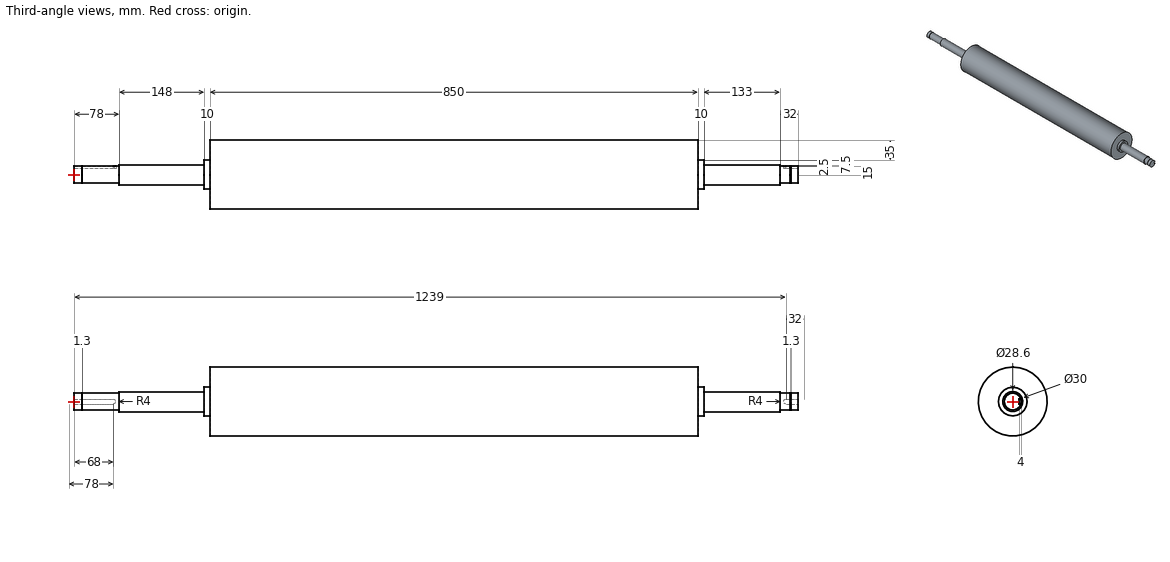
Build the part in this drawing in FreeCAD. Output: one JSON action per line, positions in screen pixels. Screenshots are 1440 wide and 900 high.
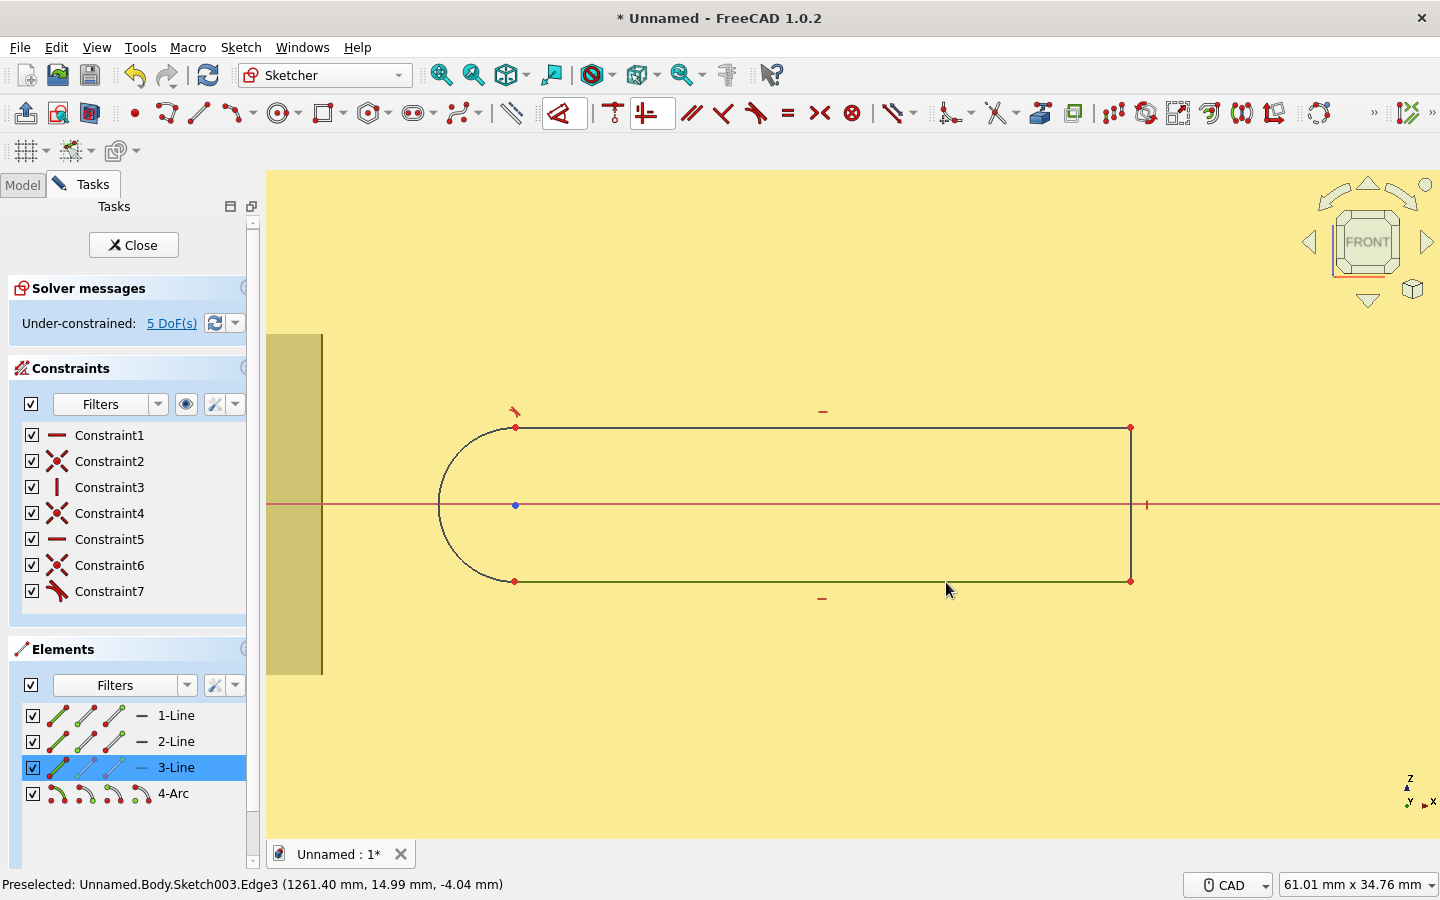
{"action": "left_click", "coordinate": [453, 460]}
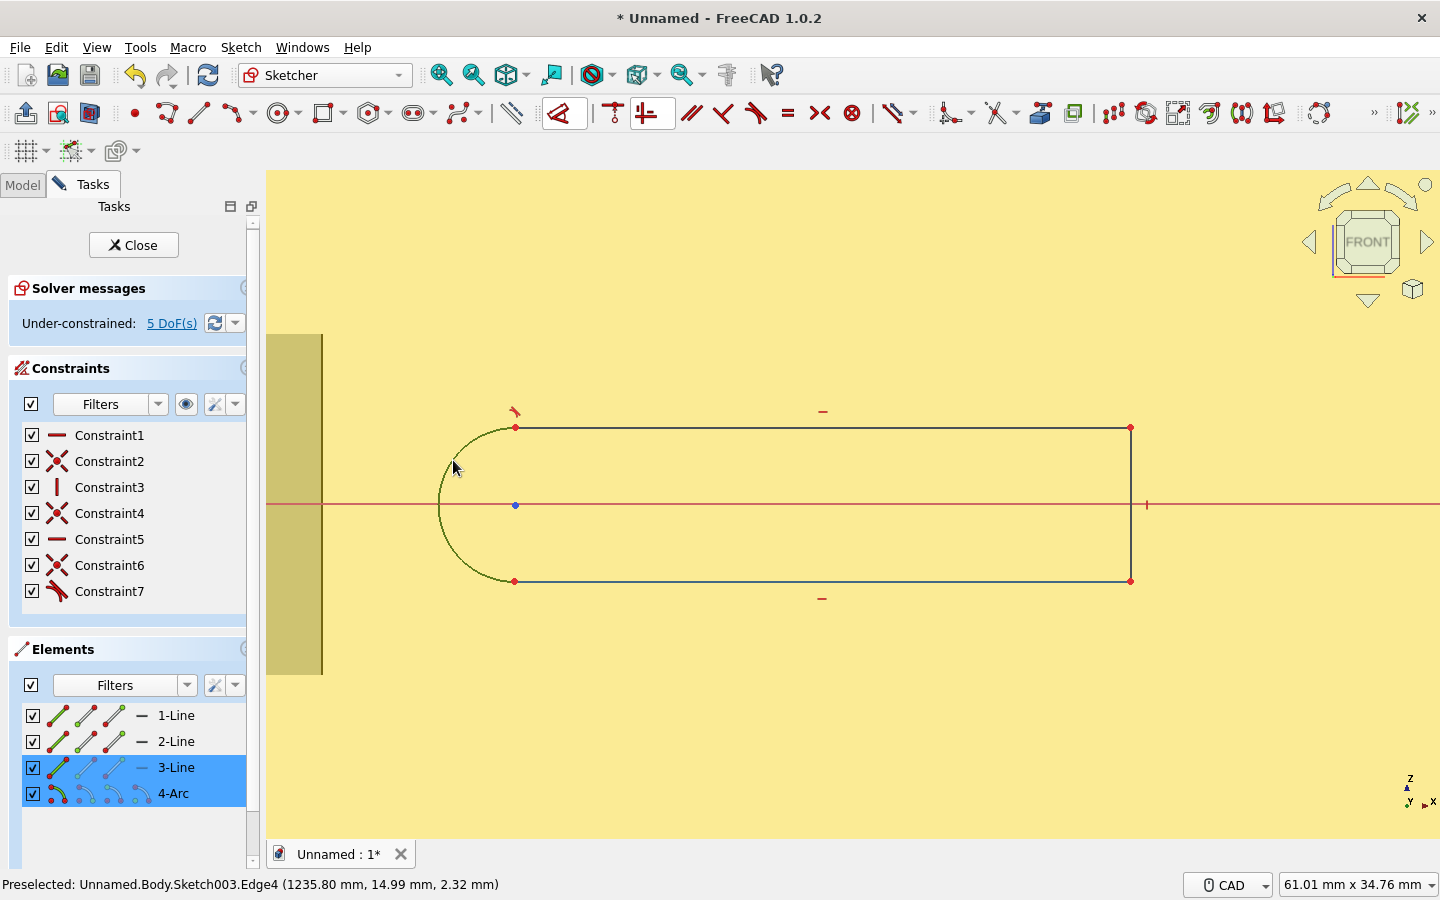
{"action": "left_click", "coordinate": [756, 114]}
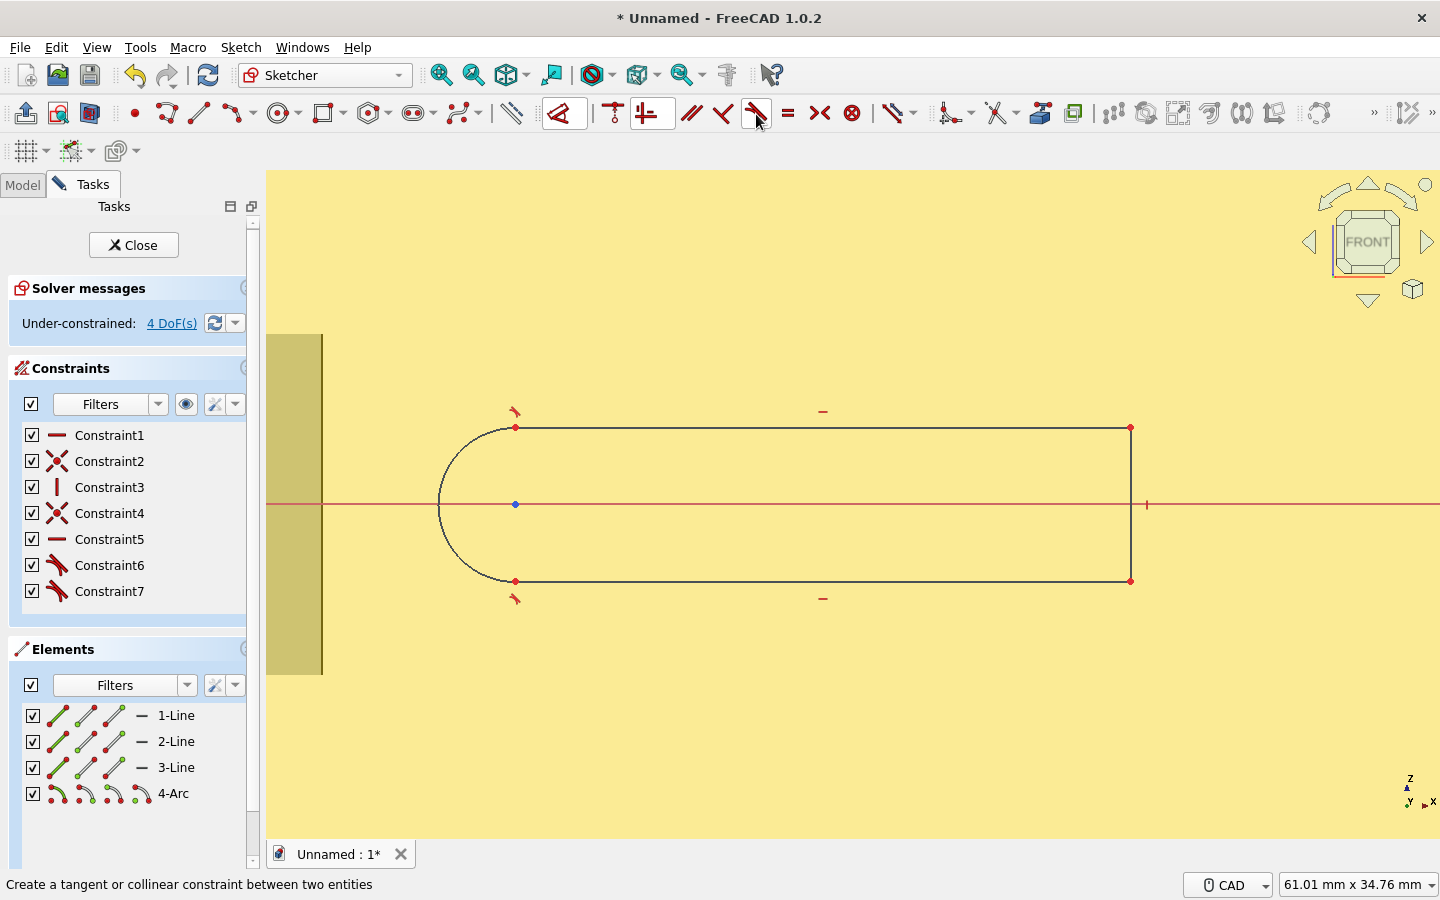
{"action": "left_click", "coordinate": [515, 505]}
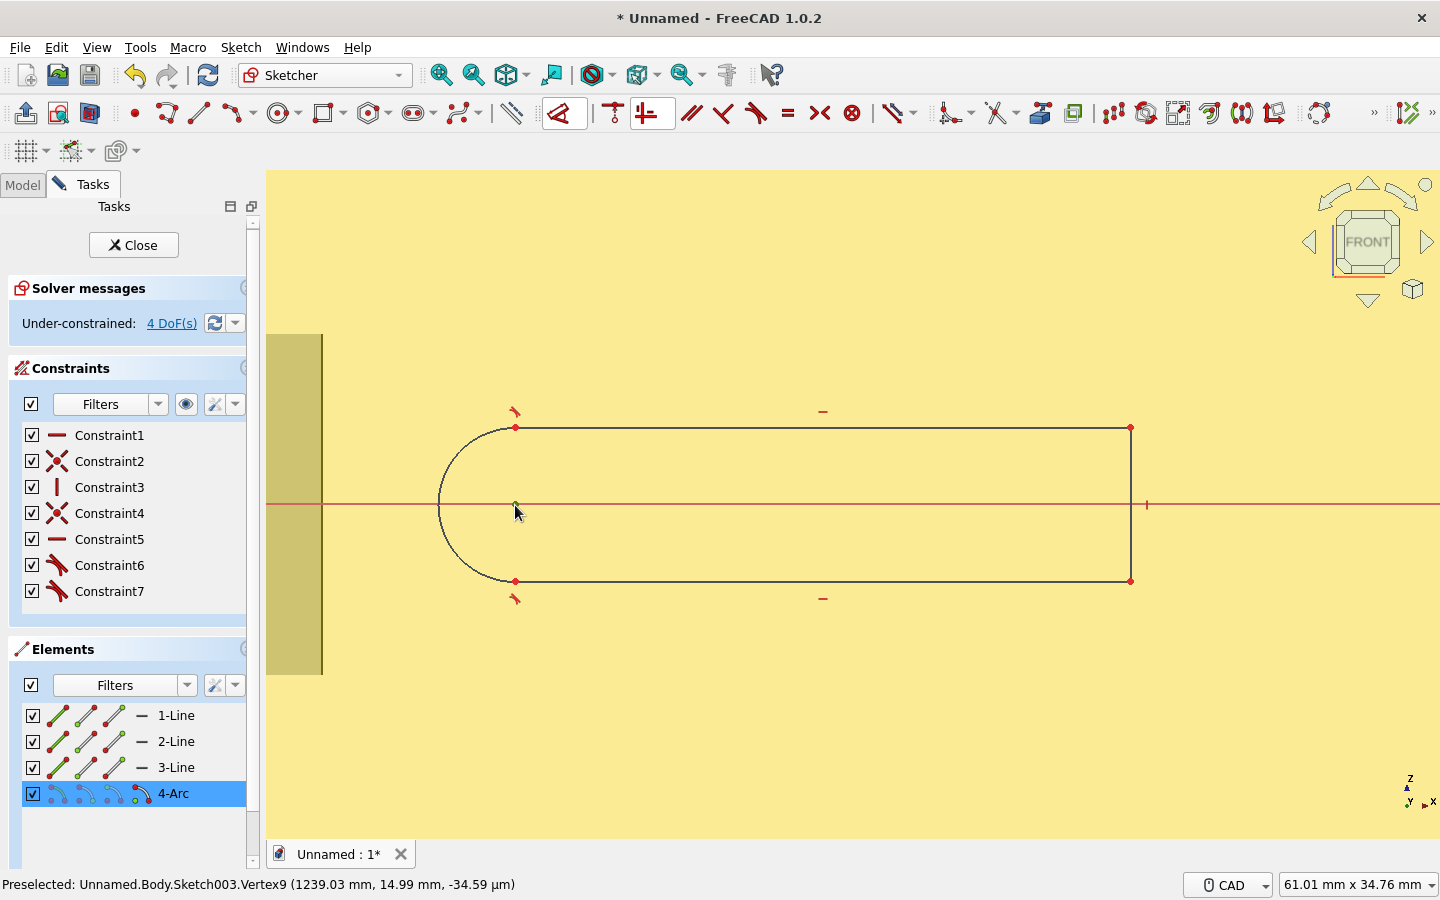
{"action": "left_click", "coordinate": [364, 504]}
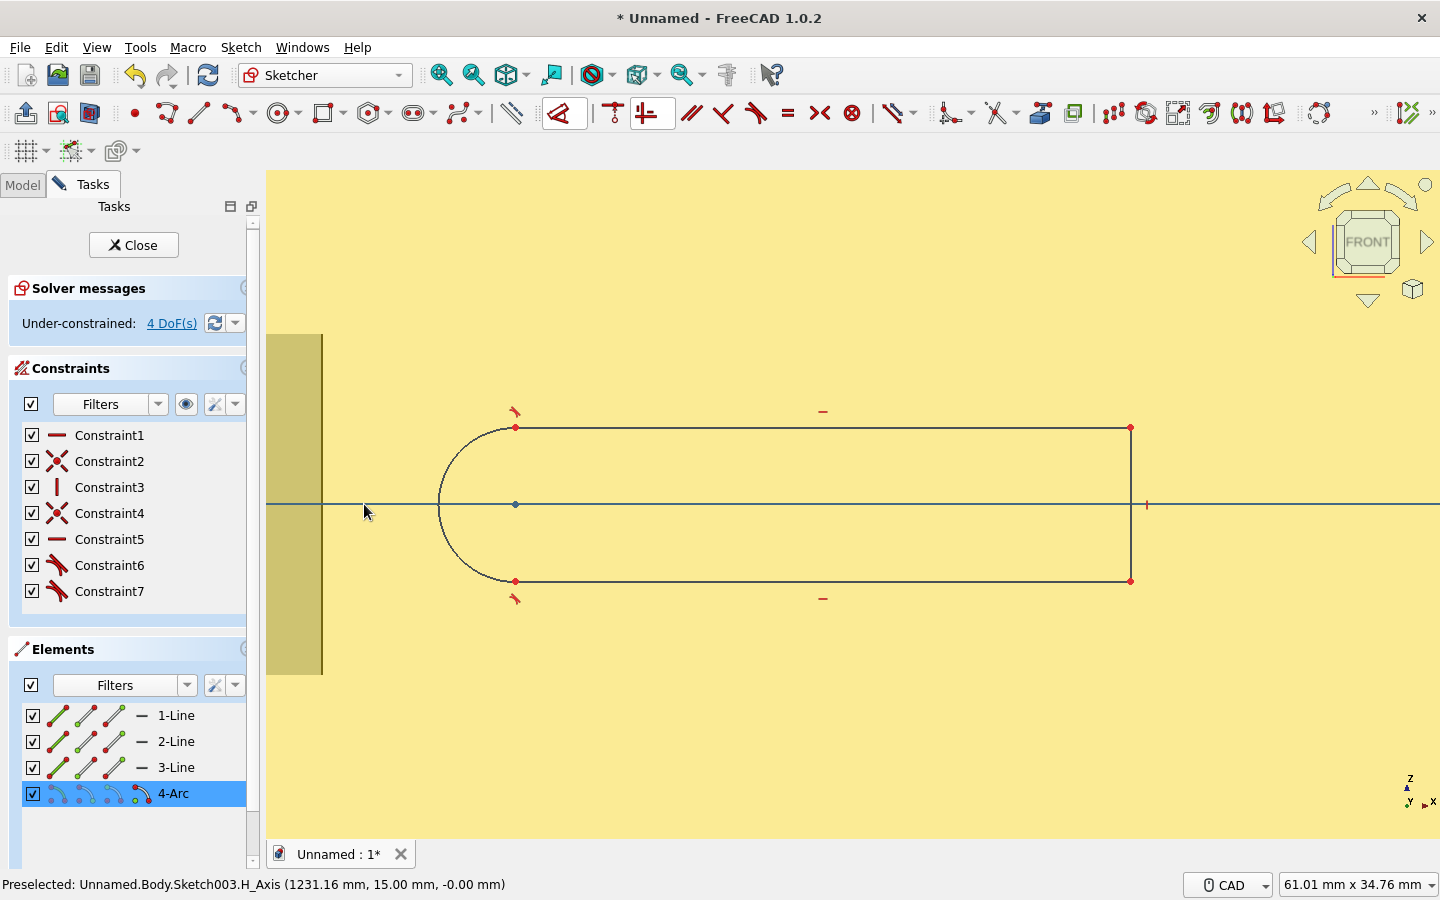
{"action": "left_click", "coordinate": [614, 114]}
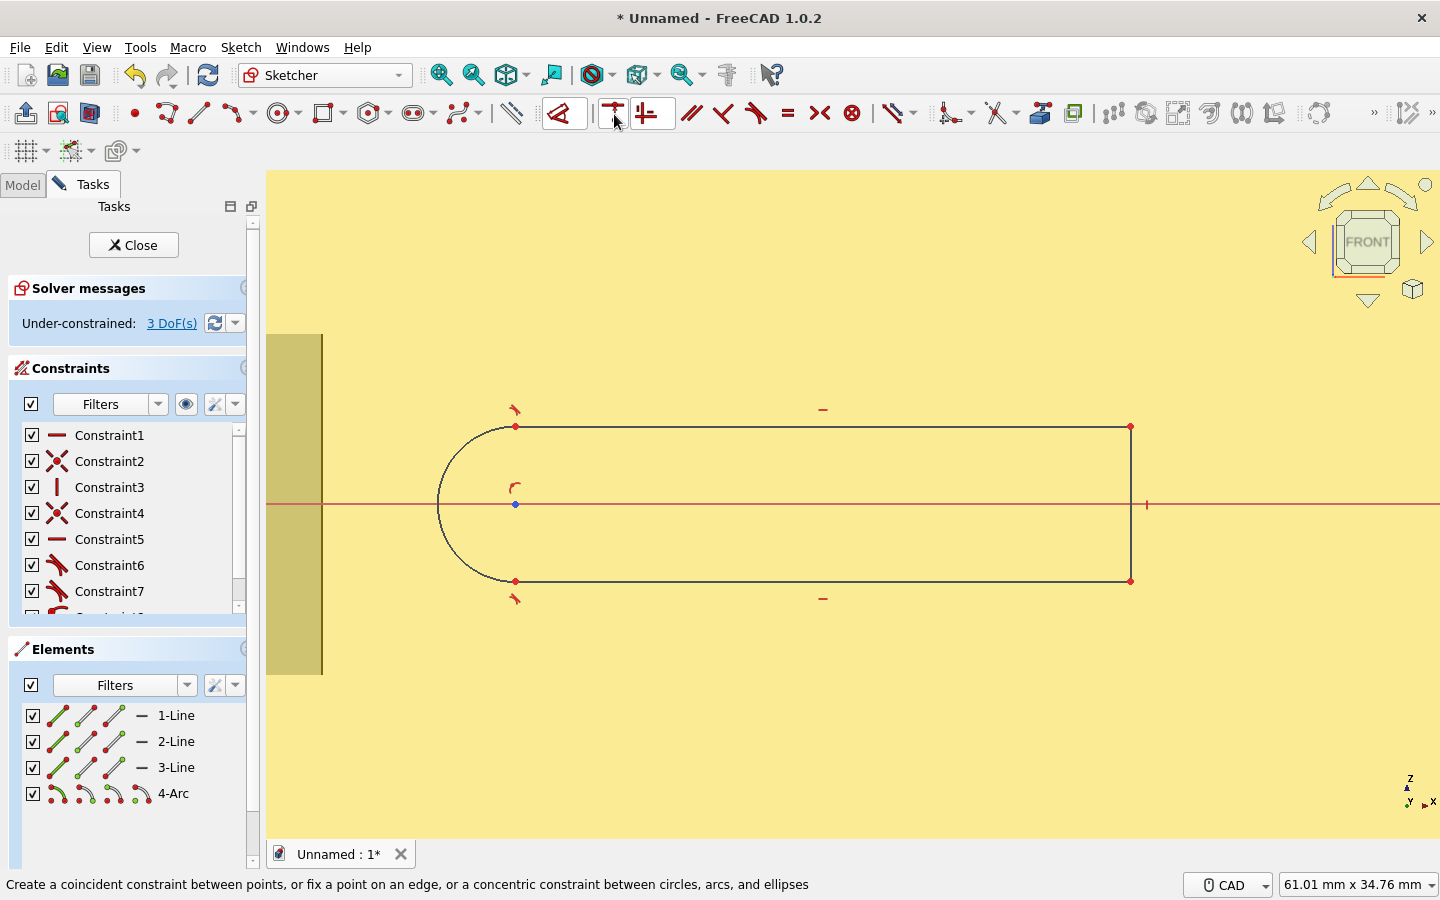
{"action": "left_click", "coordinate": [453, 459]}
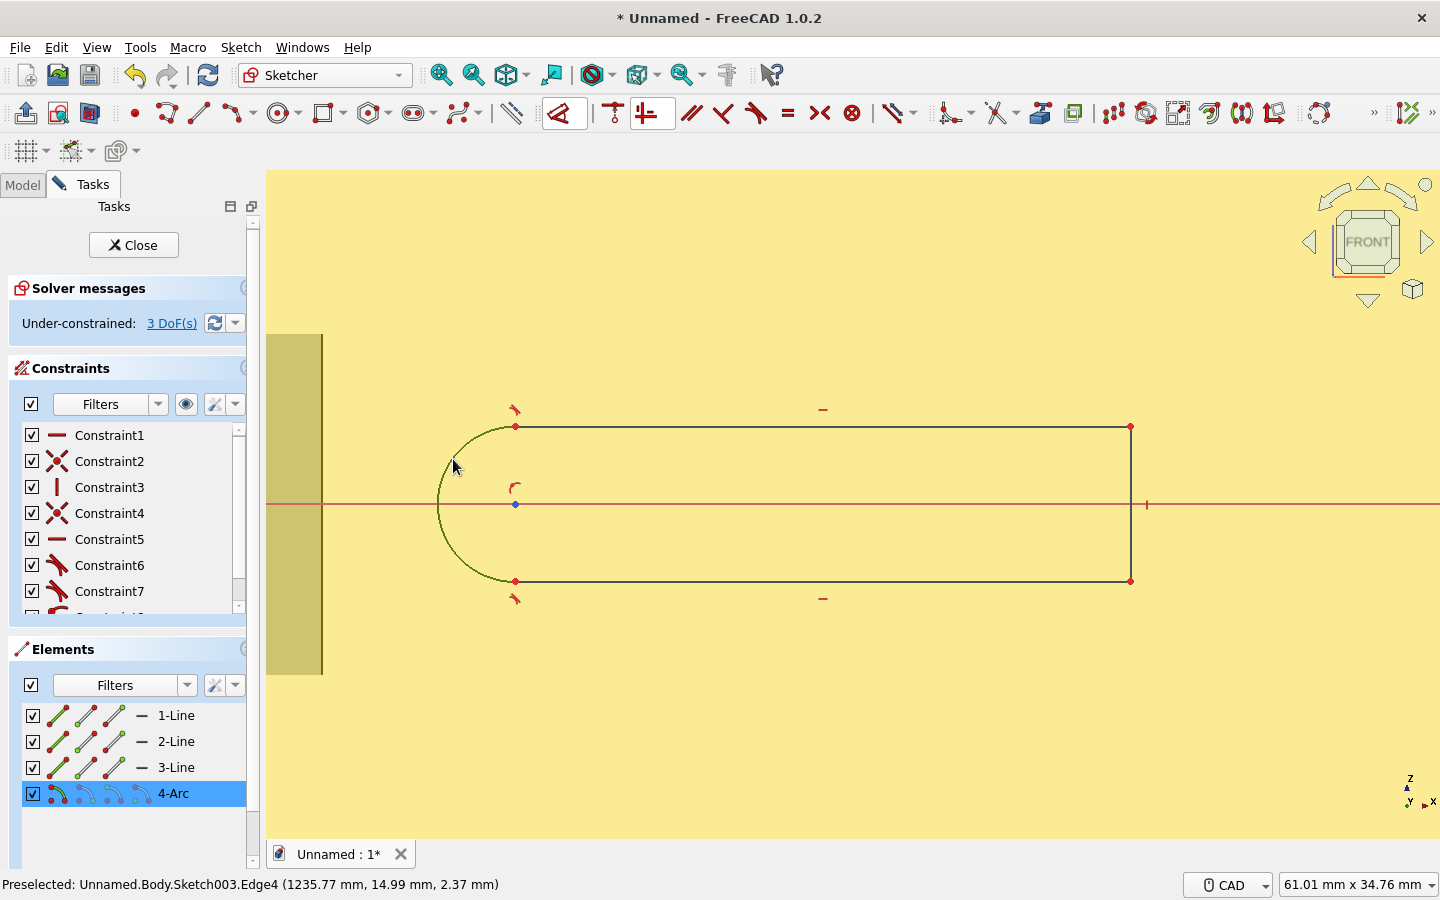
{"action": "left_click", "coordinate": [582, 114]}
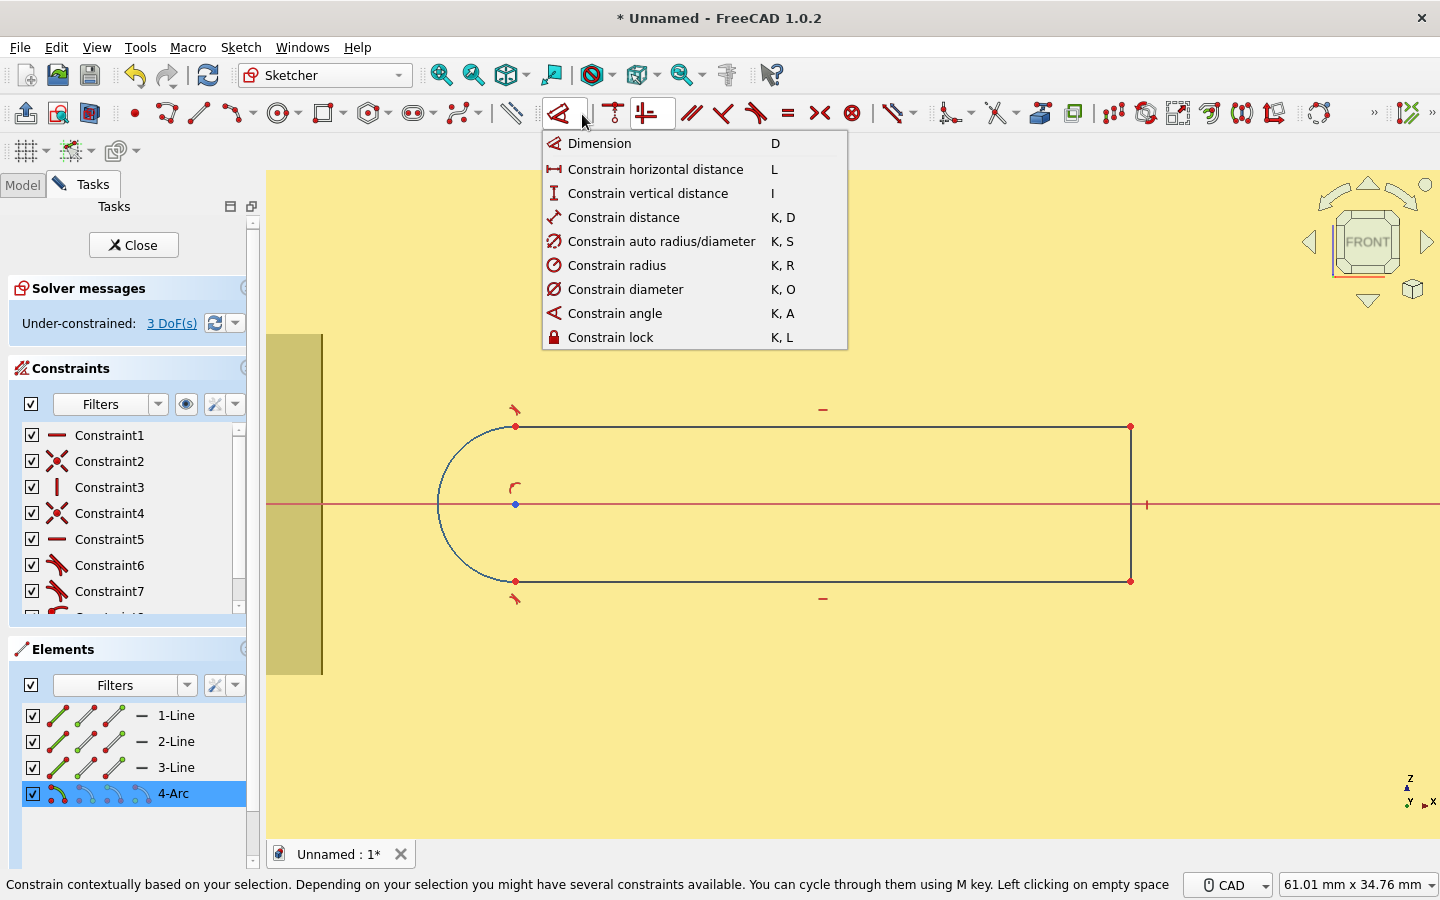
{"action": "left_click", "coordinate": [695, 265]}